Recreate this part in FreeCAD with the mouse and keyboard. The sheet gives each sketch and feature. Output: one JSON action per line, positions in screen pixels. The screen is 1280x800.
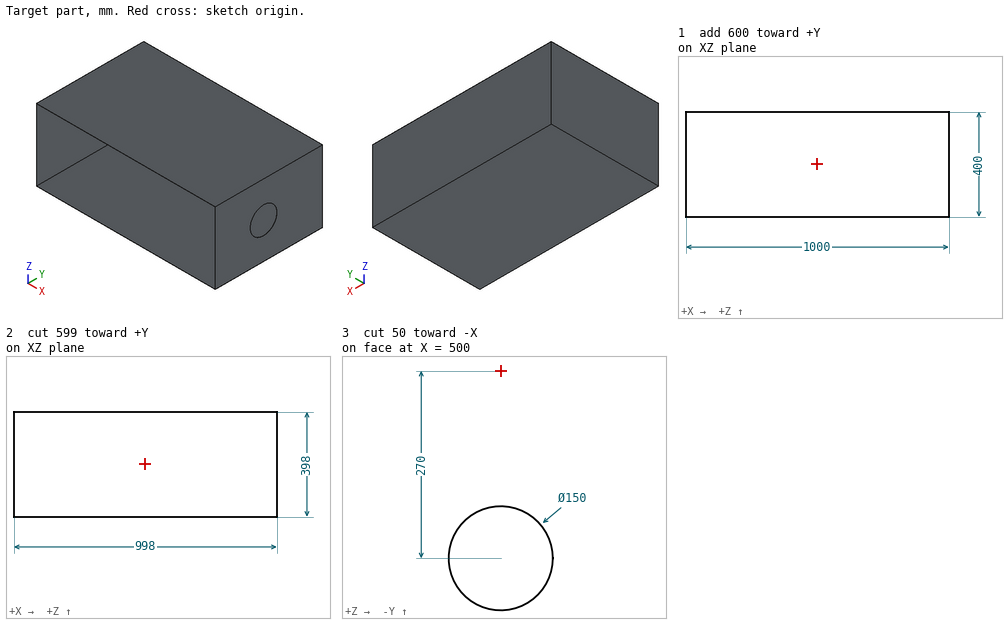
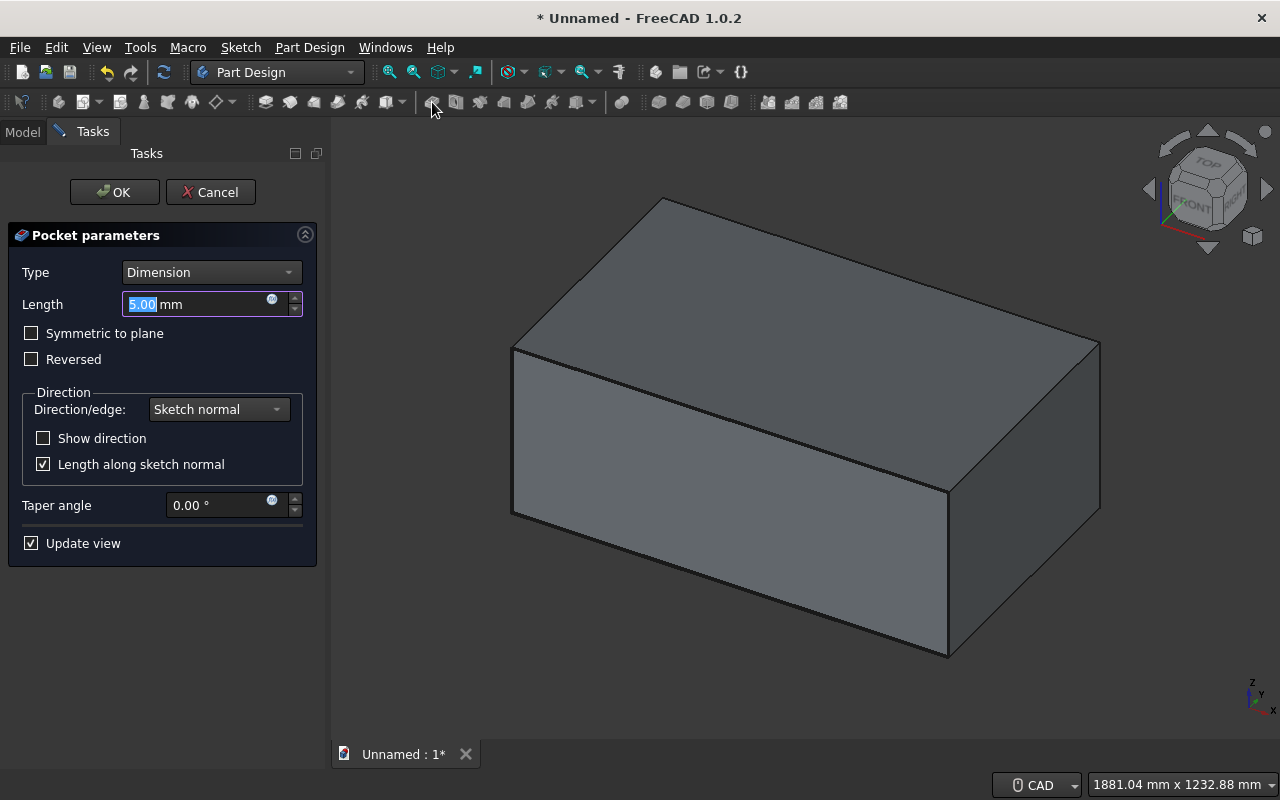
{"action": "type", "text": "599"}
{"action": "key", "text": "Tab"}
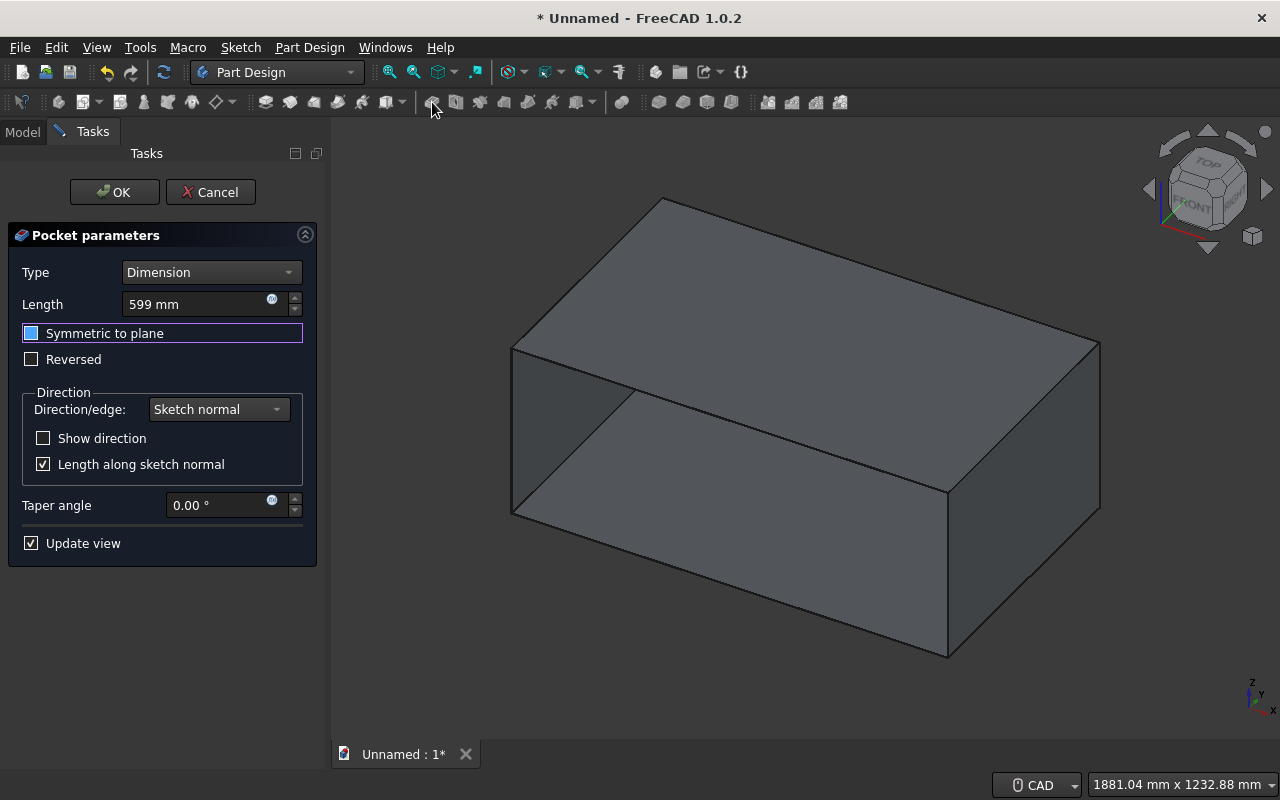
{"action": "left_click", "coordinate": [115, 192]}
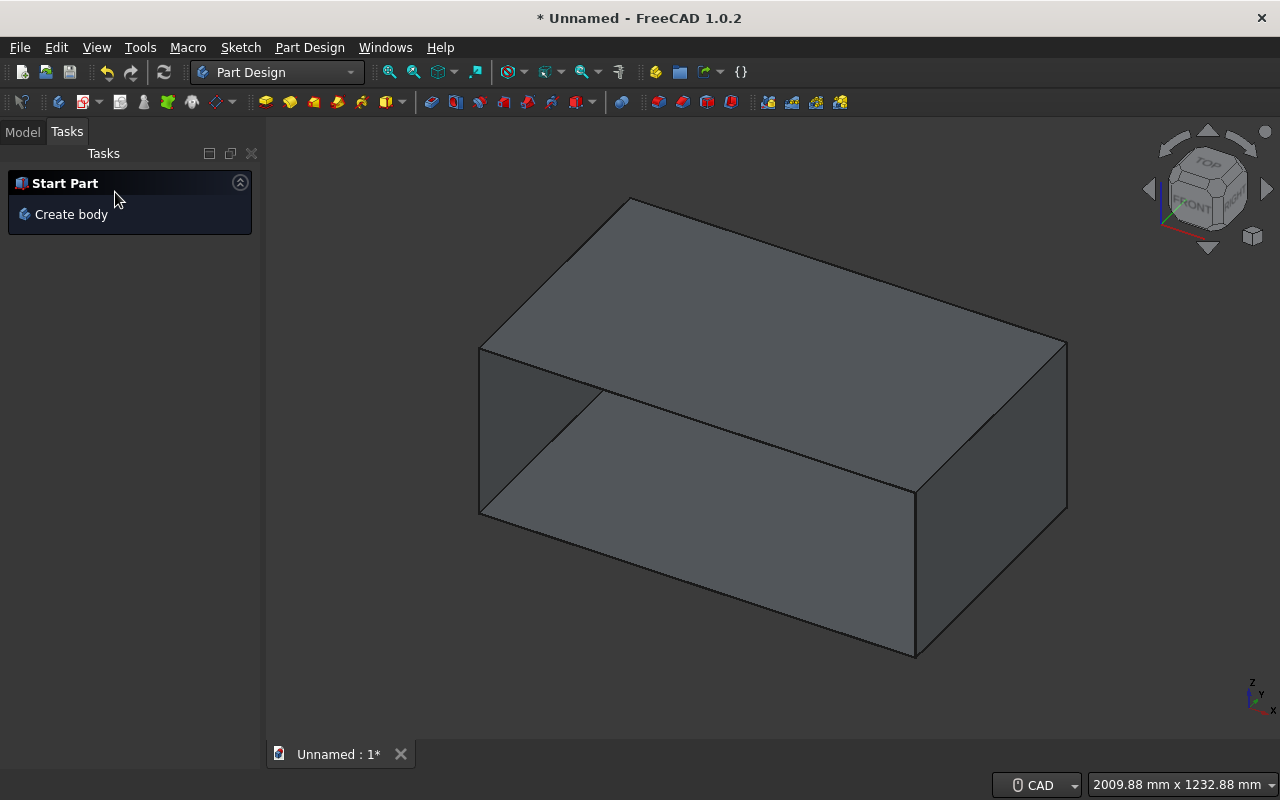
{"action": "left_click", "coordinate": [1013, 478]}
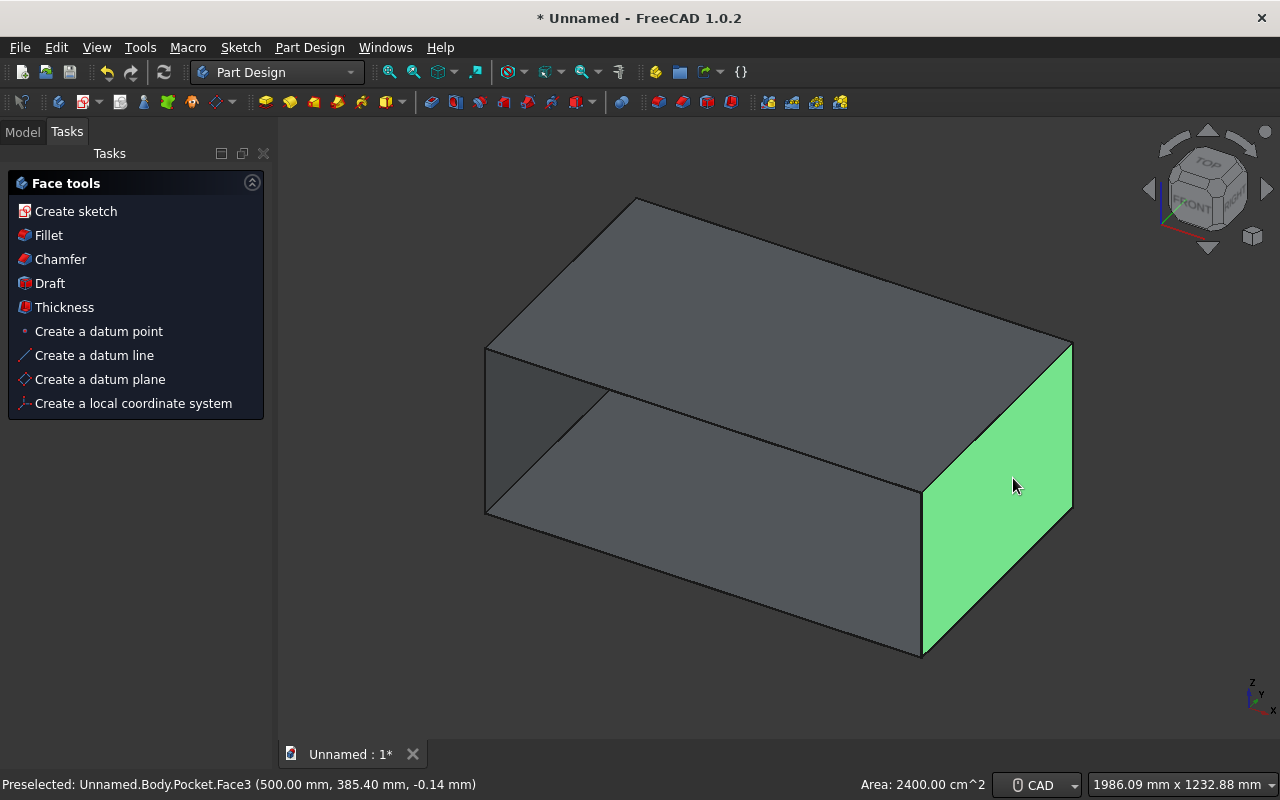
{"action": "left_click", "coordinate": [84, 102]}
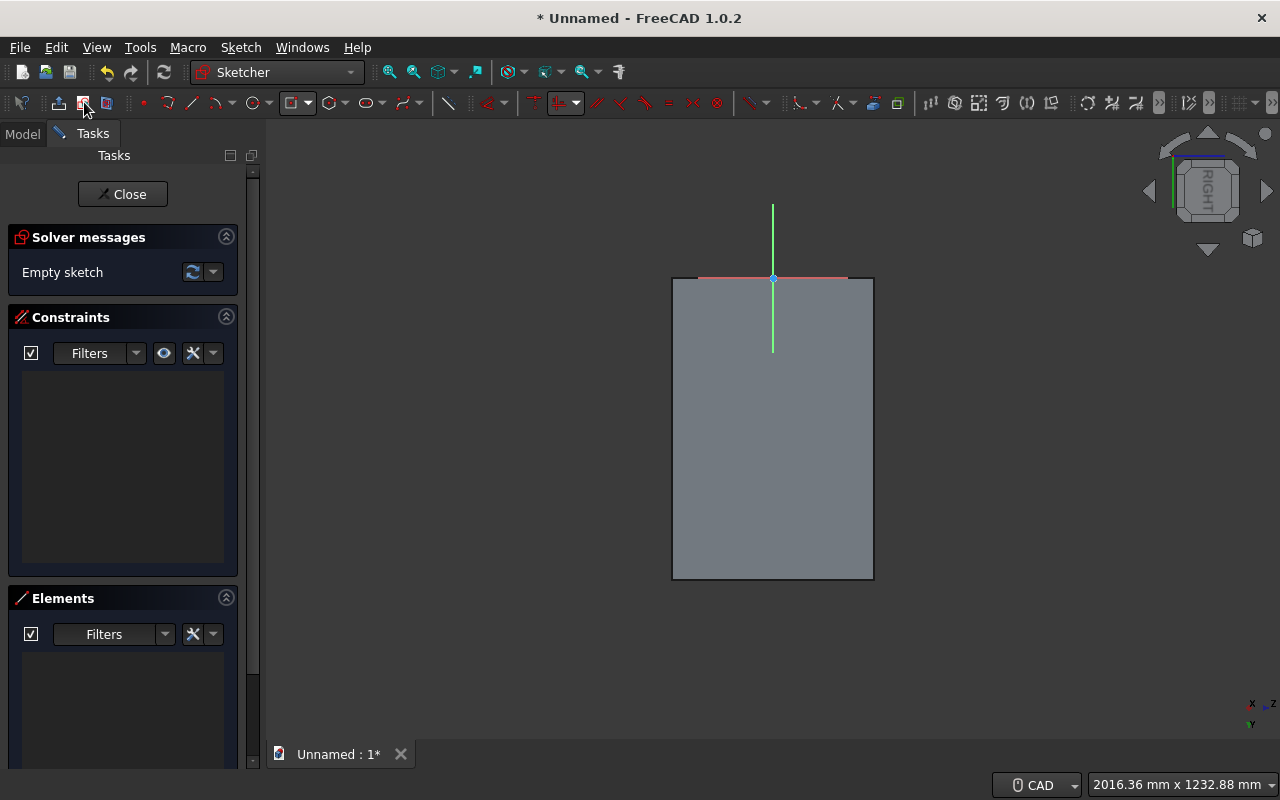
{"action": "scroll", "coordinate": [829, 313], "scroll_direction": "up", "scroll_amount": 4}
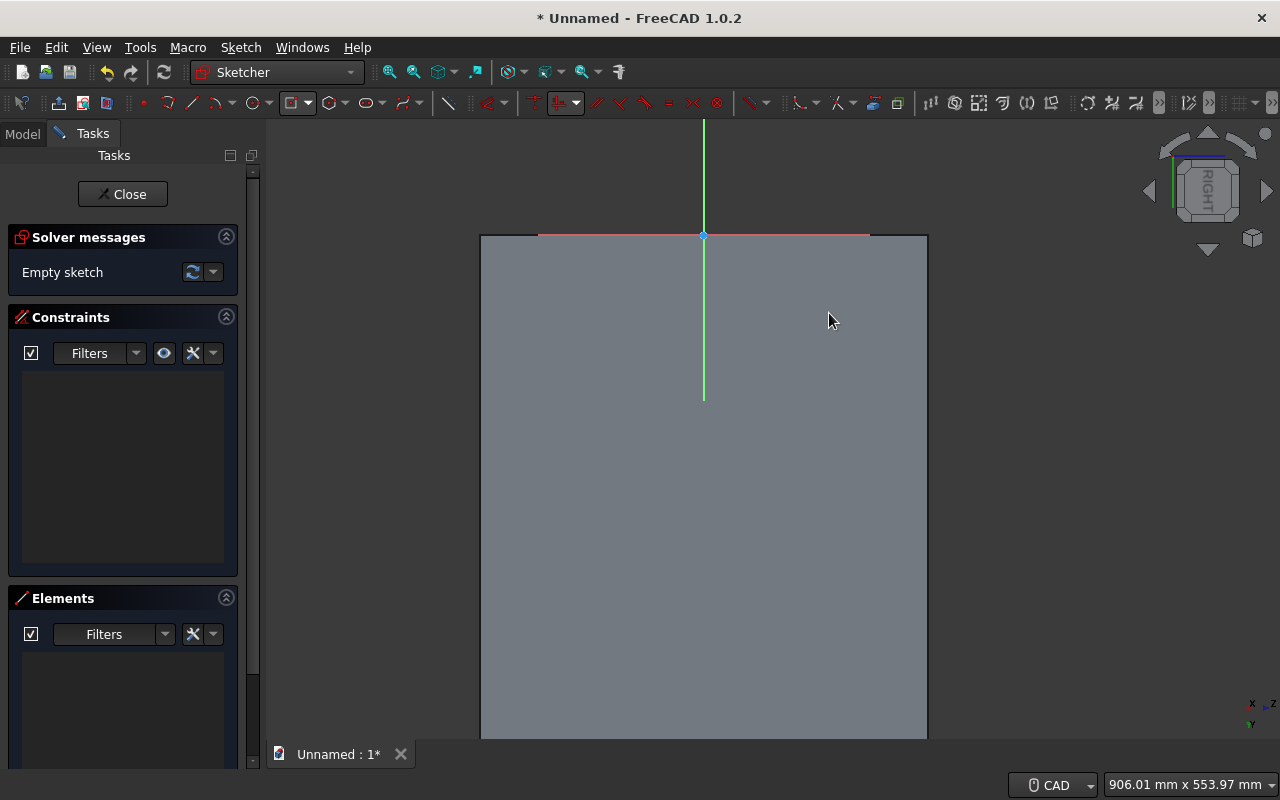
{"action": "key", "text": "g c"}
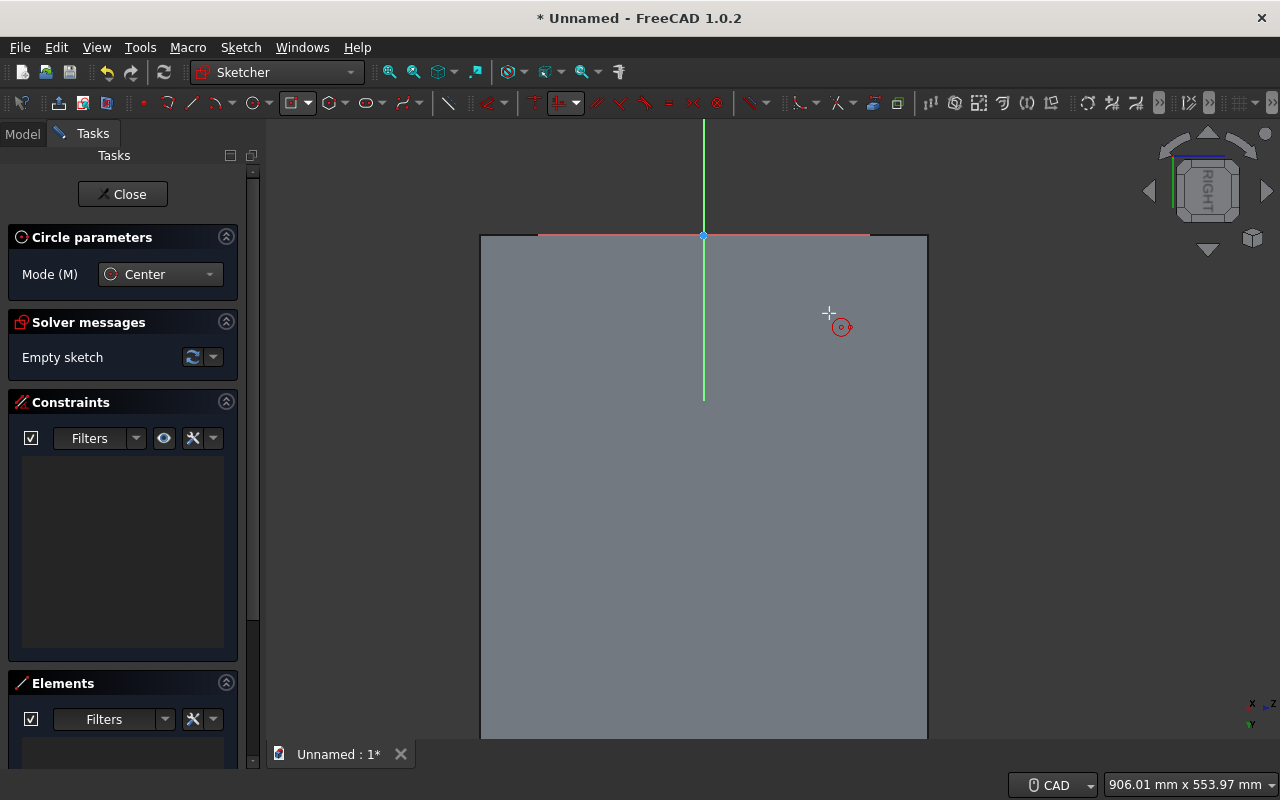
{"action": "left_click", "coordinate": [704, 537]}
{"action": "left_click", "coordinate": [763, 478]}
{"action": "key", "text": "Escape"}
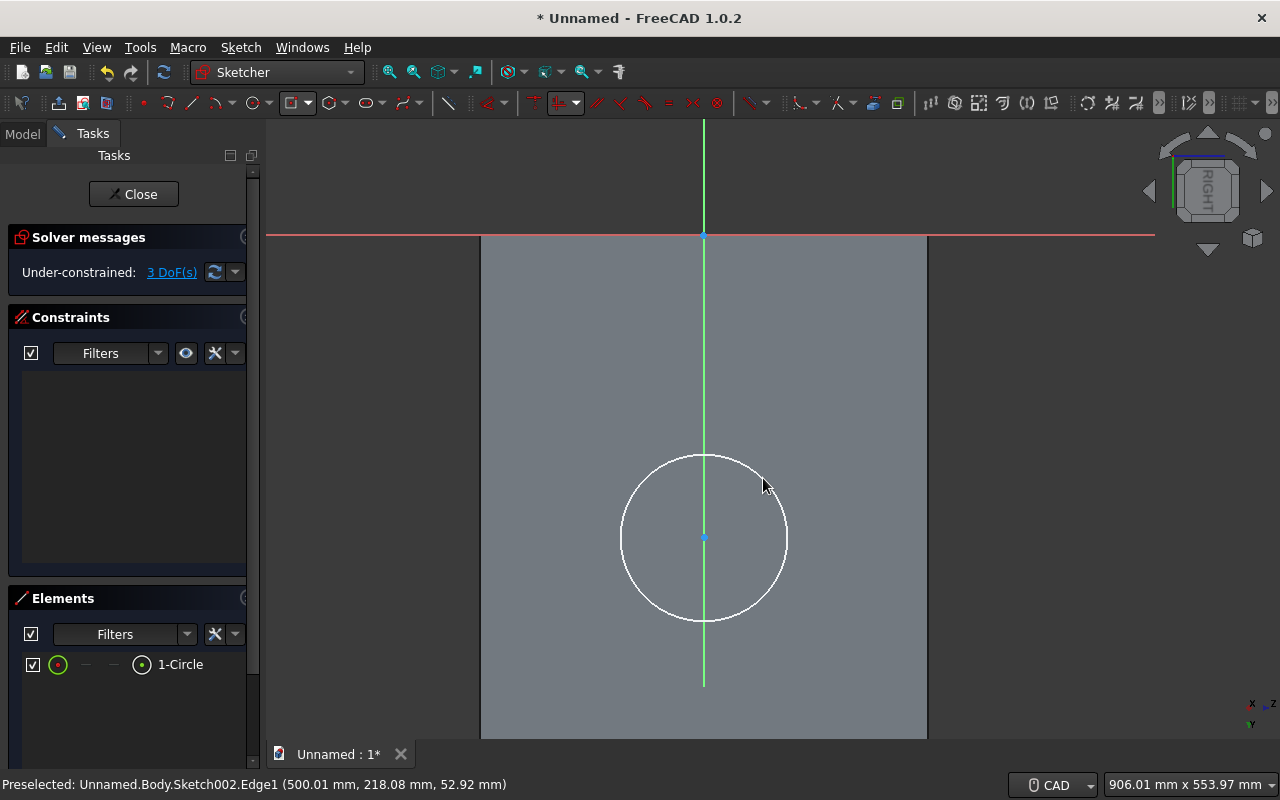
{"action": "left_click", "coordinate": [704, 538]}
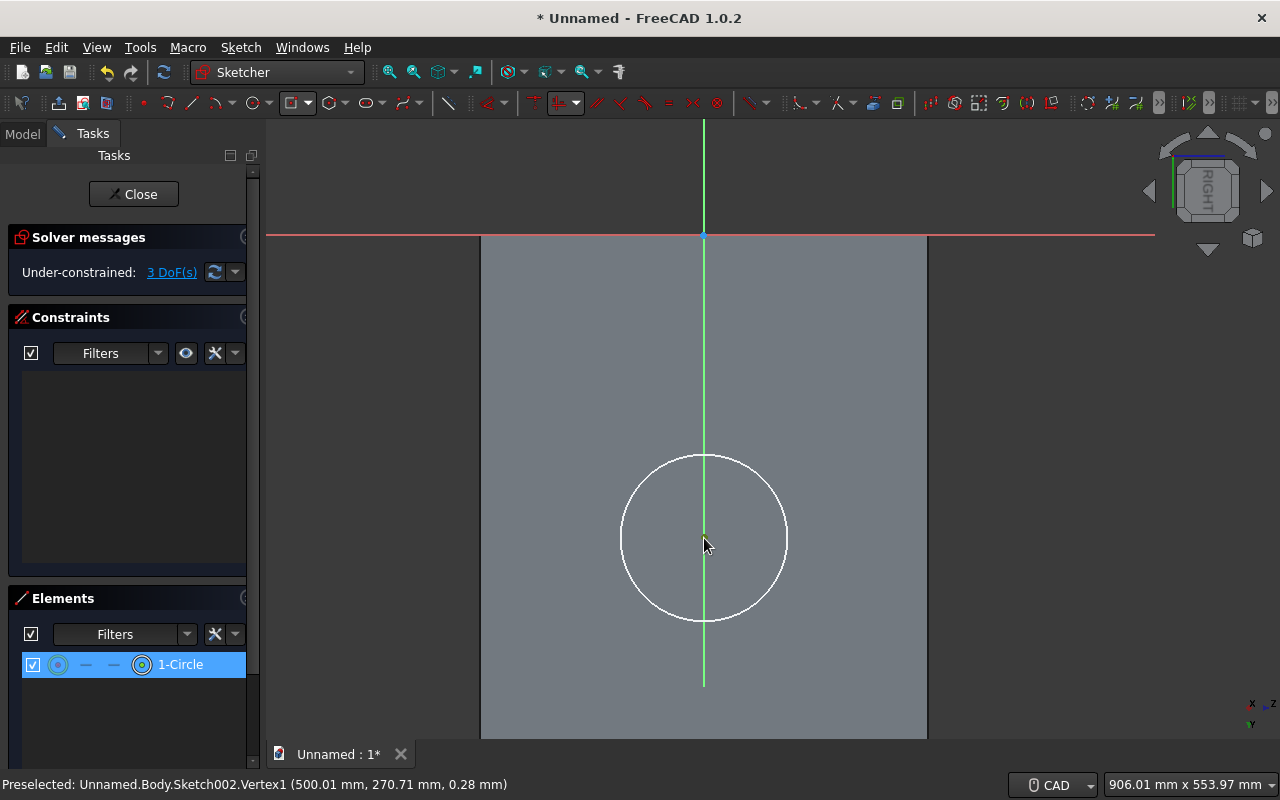
{"action": "left_click", "coordinate": [704, 671]}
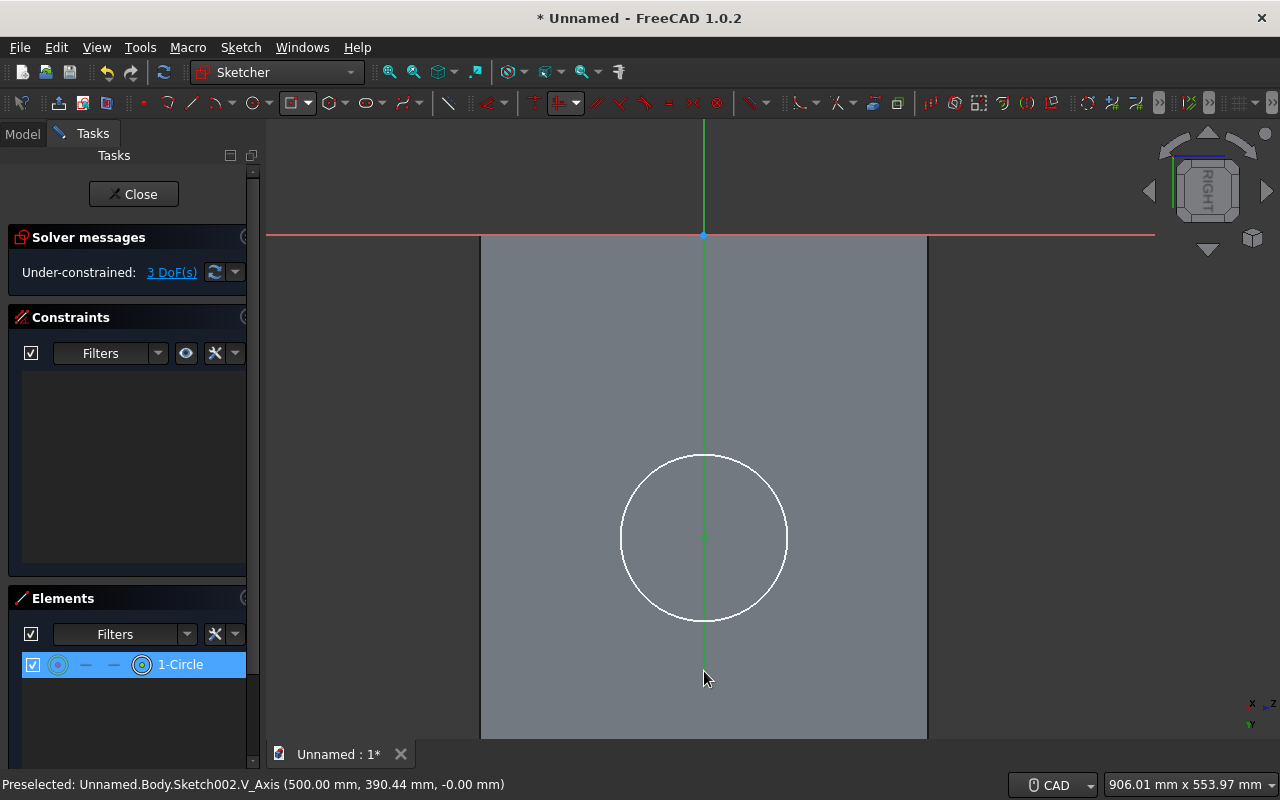
{"action": "key", "text": "c"}